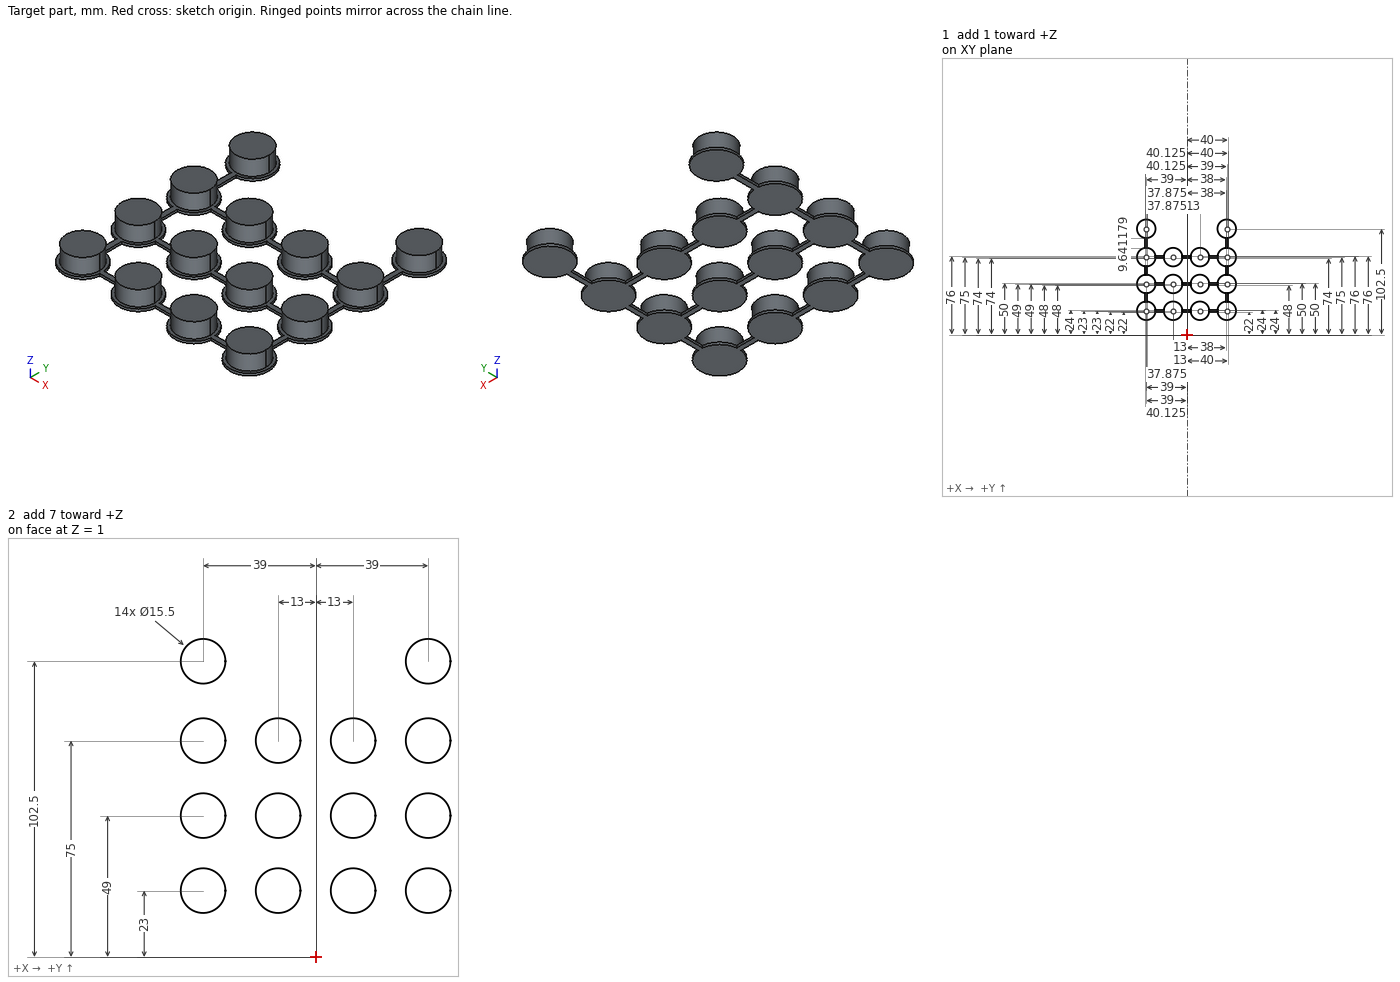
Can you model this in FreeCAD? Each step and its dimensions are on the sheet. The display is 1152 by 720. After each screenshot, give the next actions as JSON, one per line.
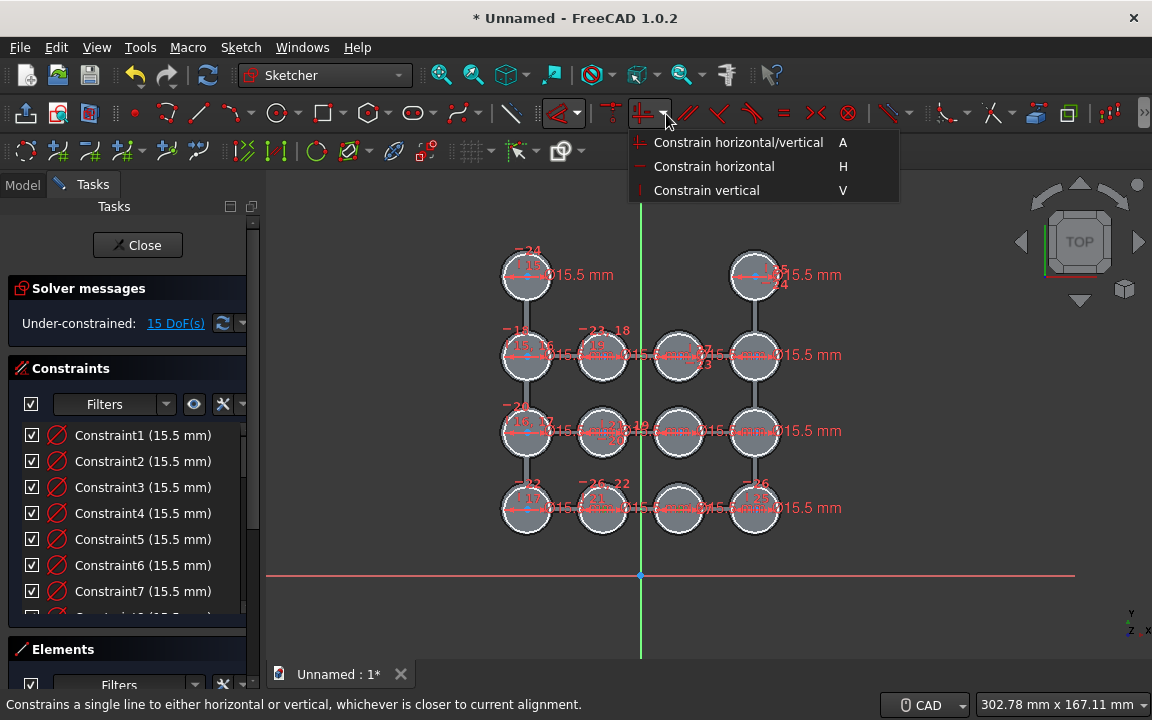
{"action": "left_click", "coordinate": [764, 166]}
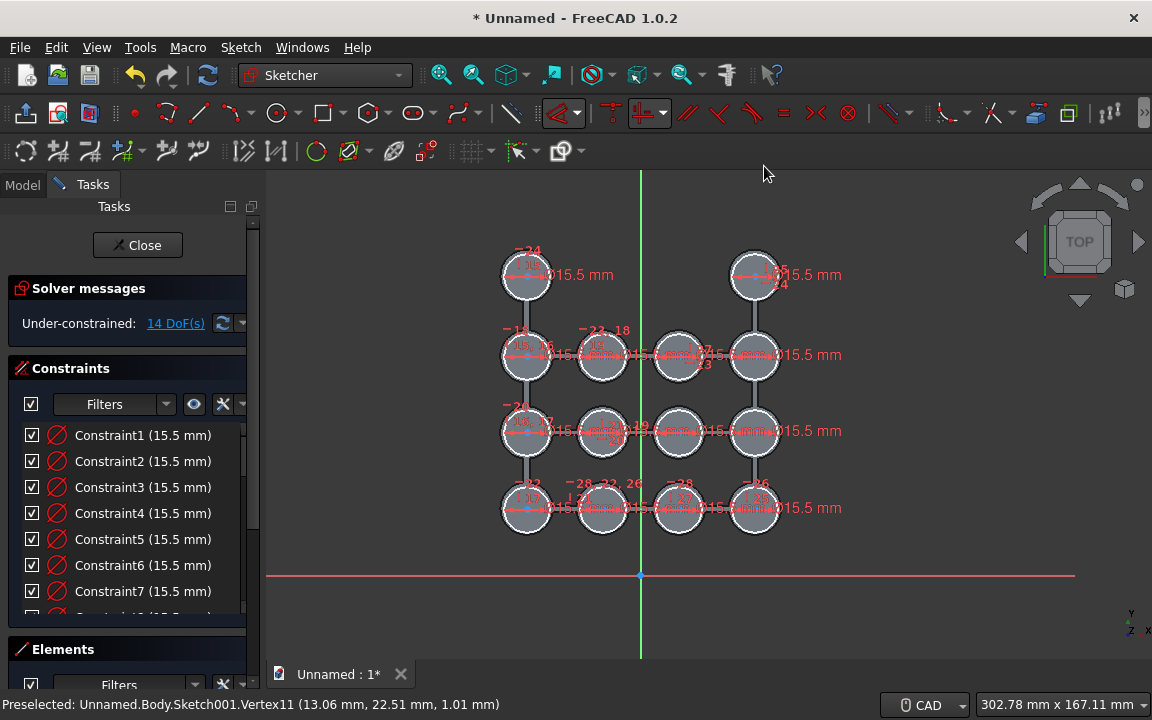
{"action": "left_click", "coordinate": [755, 510]}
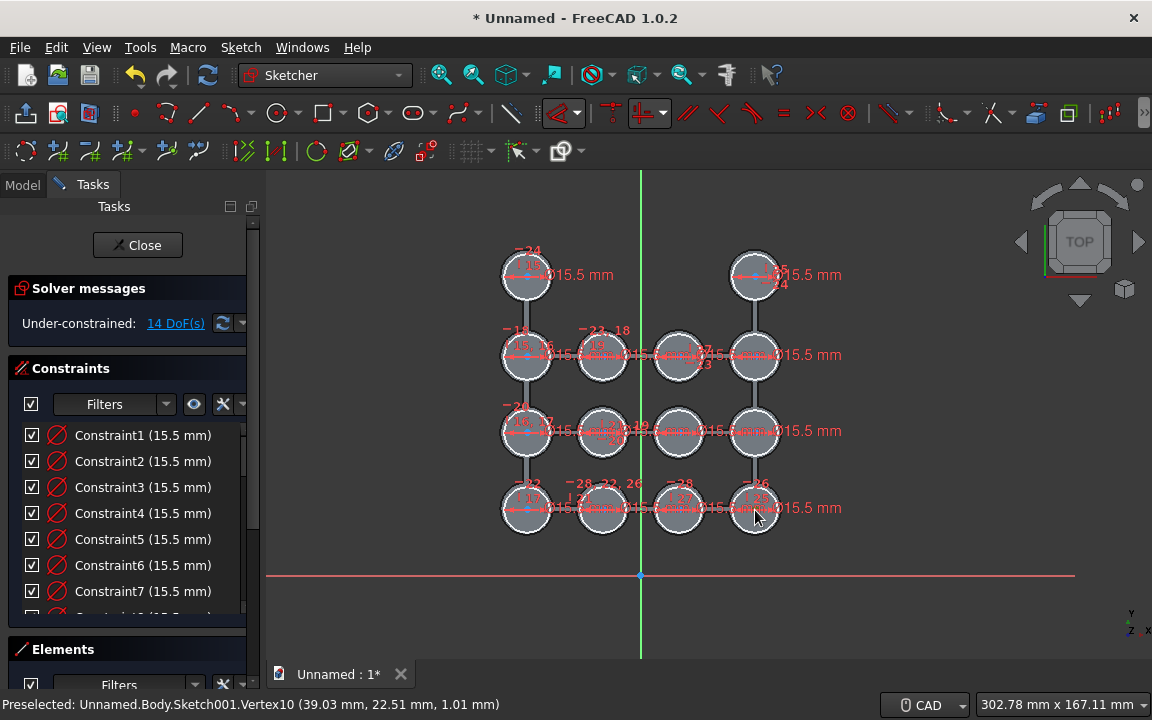
{"action": "left_click", "coordinate": [755, 433]}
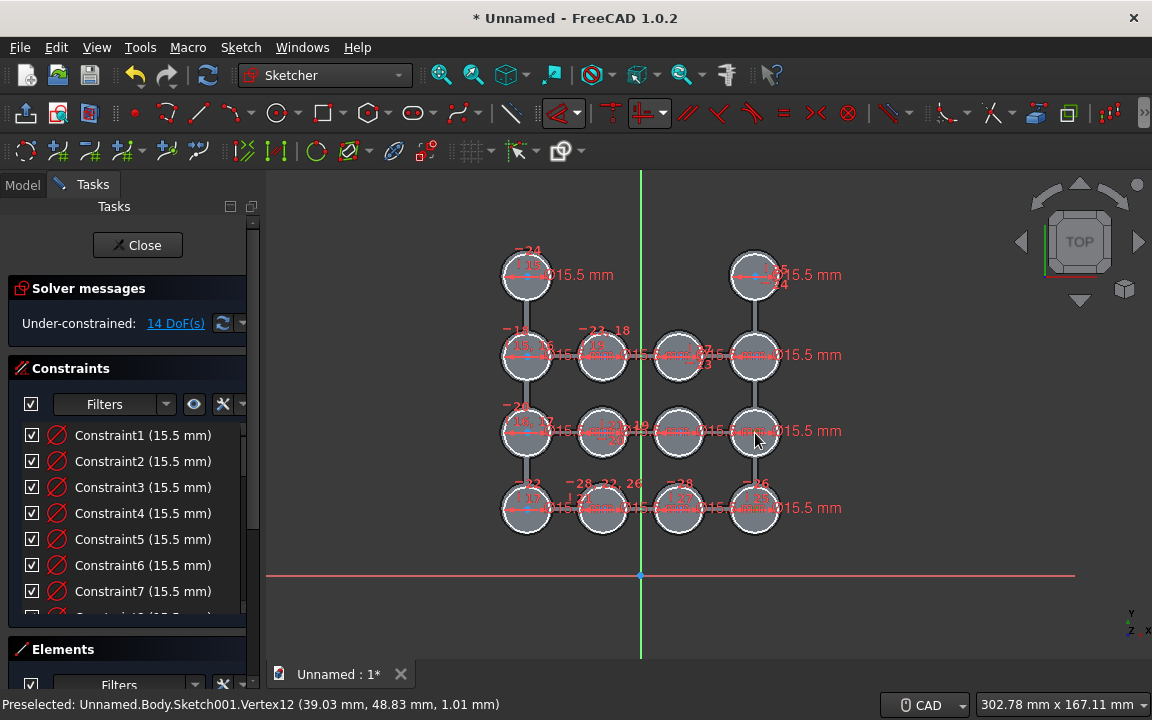
{"action": "left_click", "coordinate": [666, 114]}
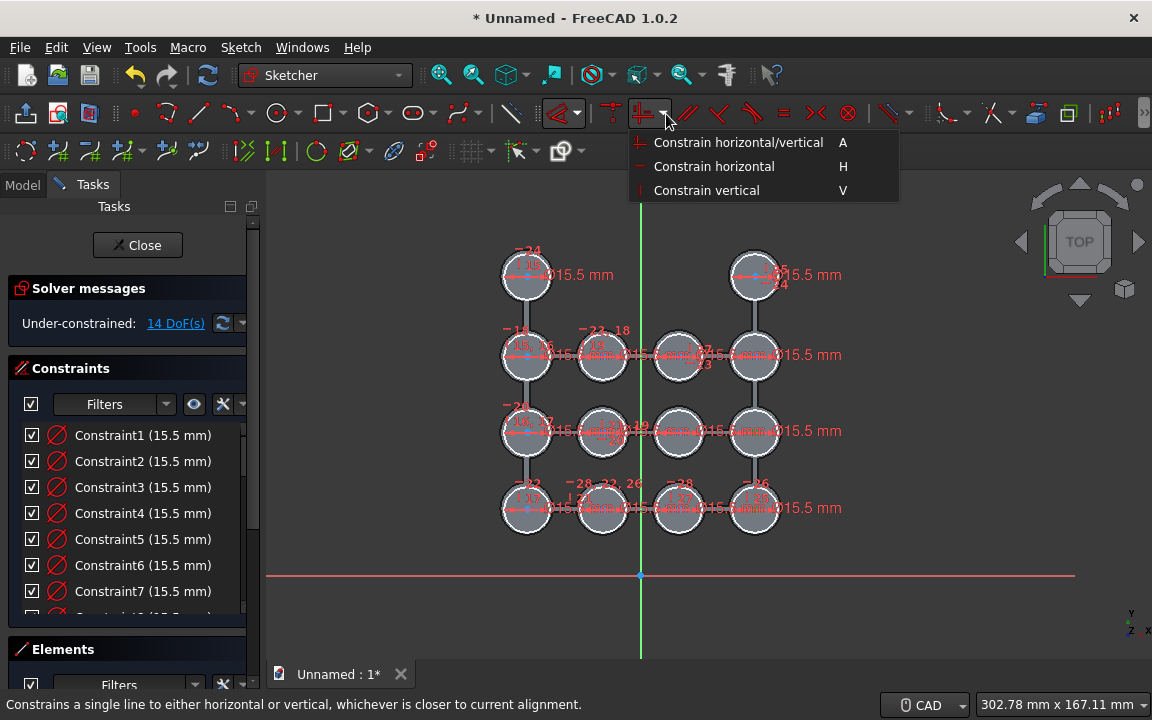
{"action": "left_click", "coordinate": [764, 190]}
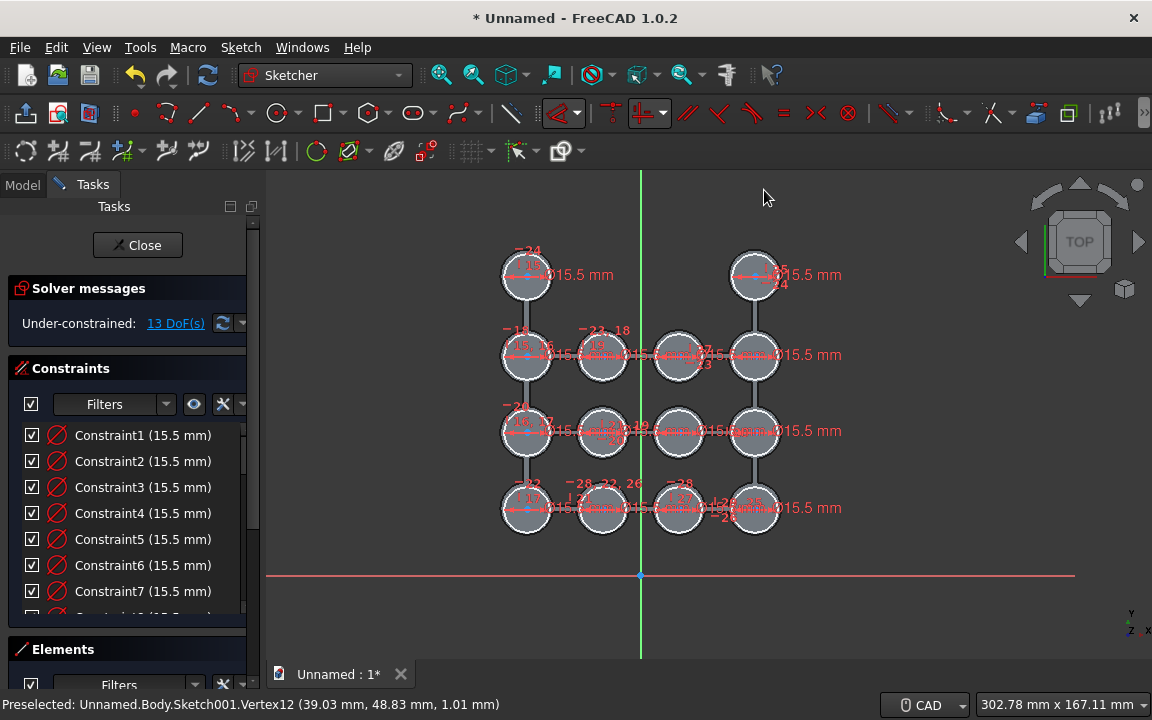
{"action": "left_click", "coordinate": [603, 433]}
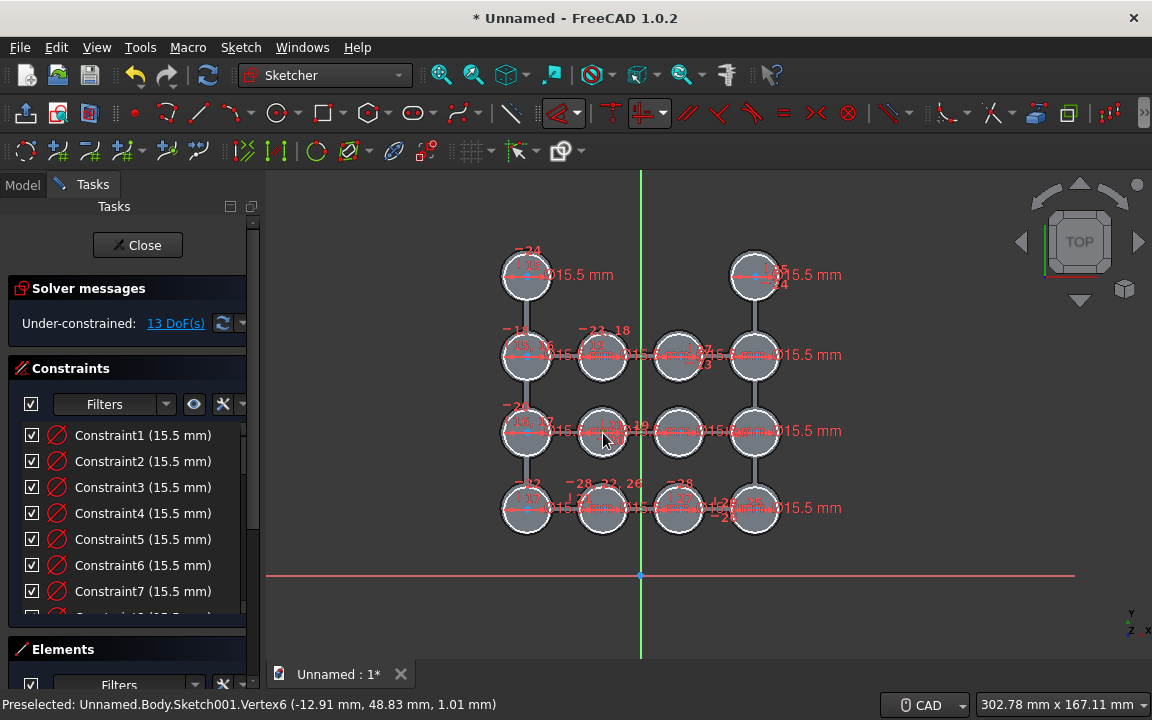
{"action": "left_click", "coordinate": [755, 433]}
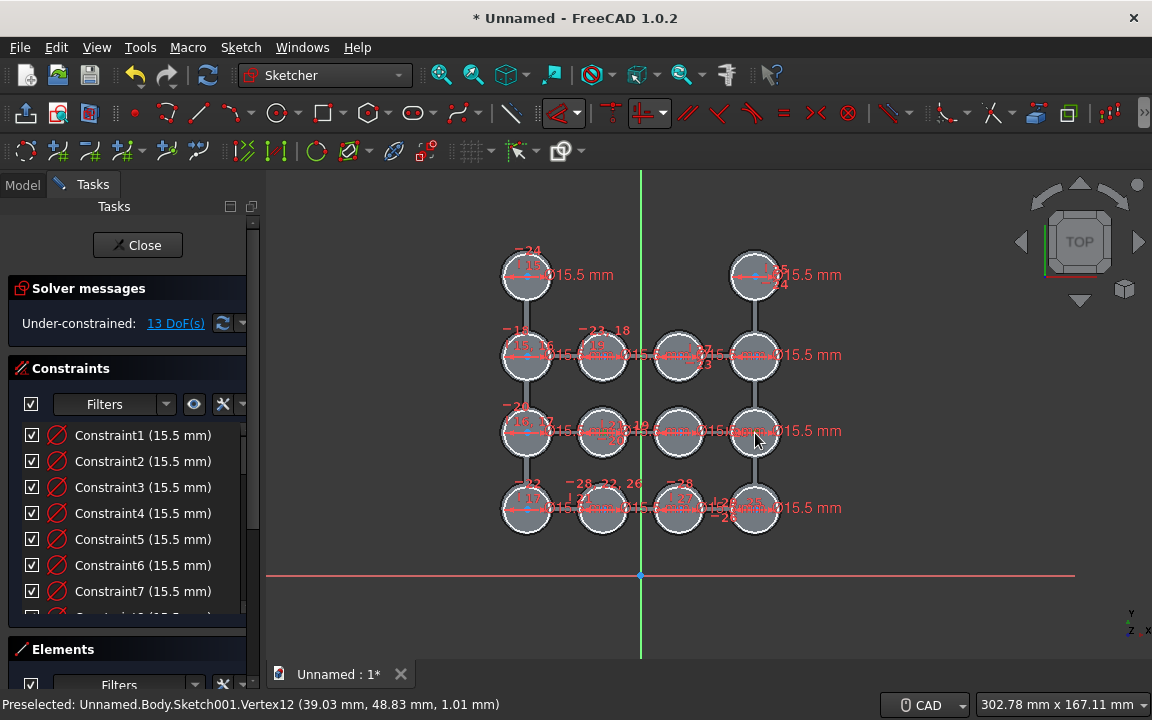
{"action": "key", "text": "h"}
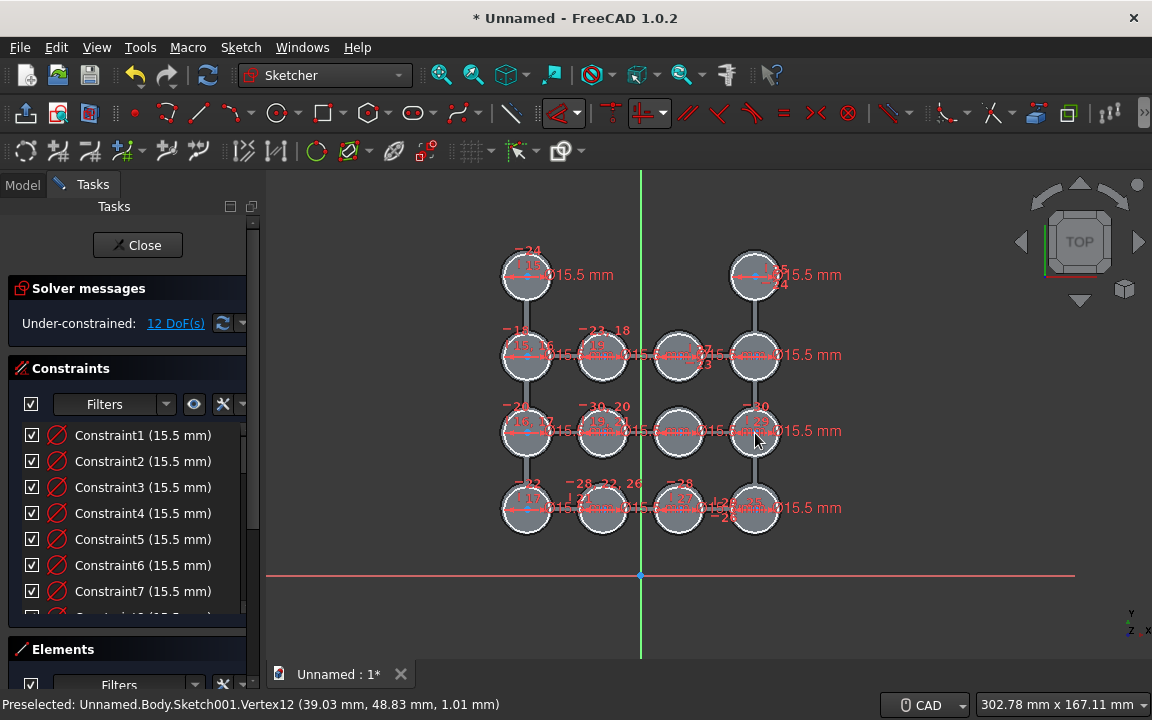
{"action": "left_click", "coordinate": [679, 357]}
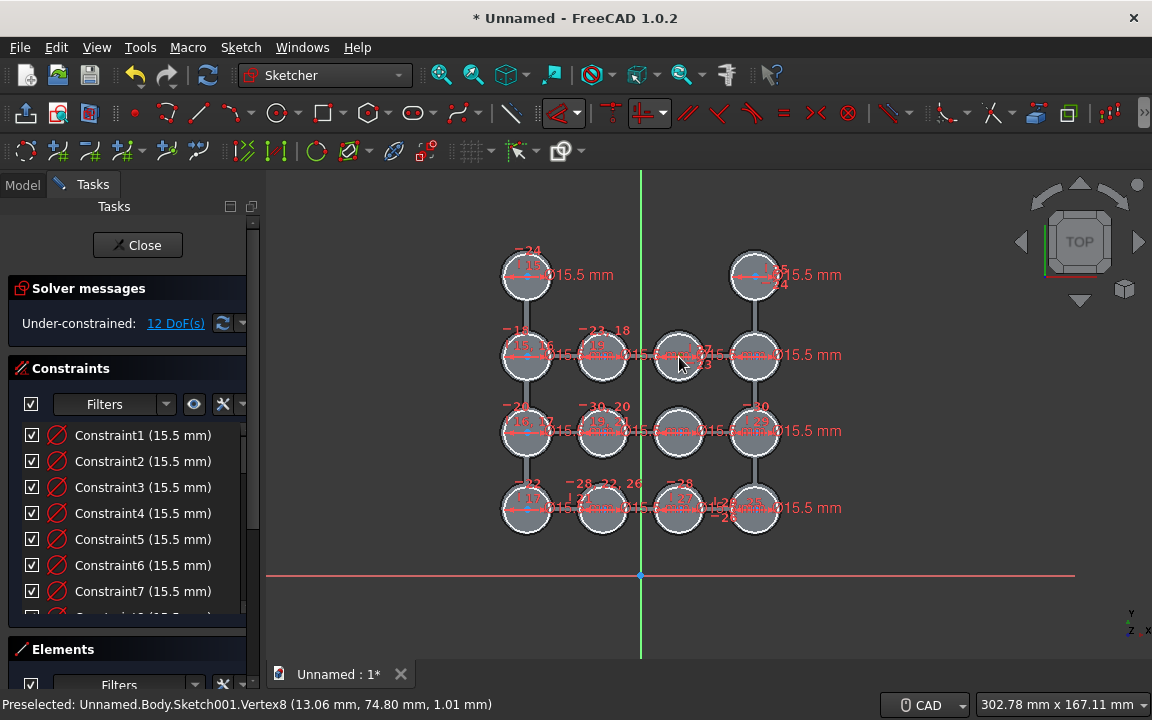
{"action": "left_click", "coordinate": [679, 433]}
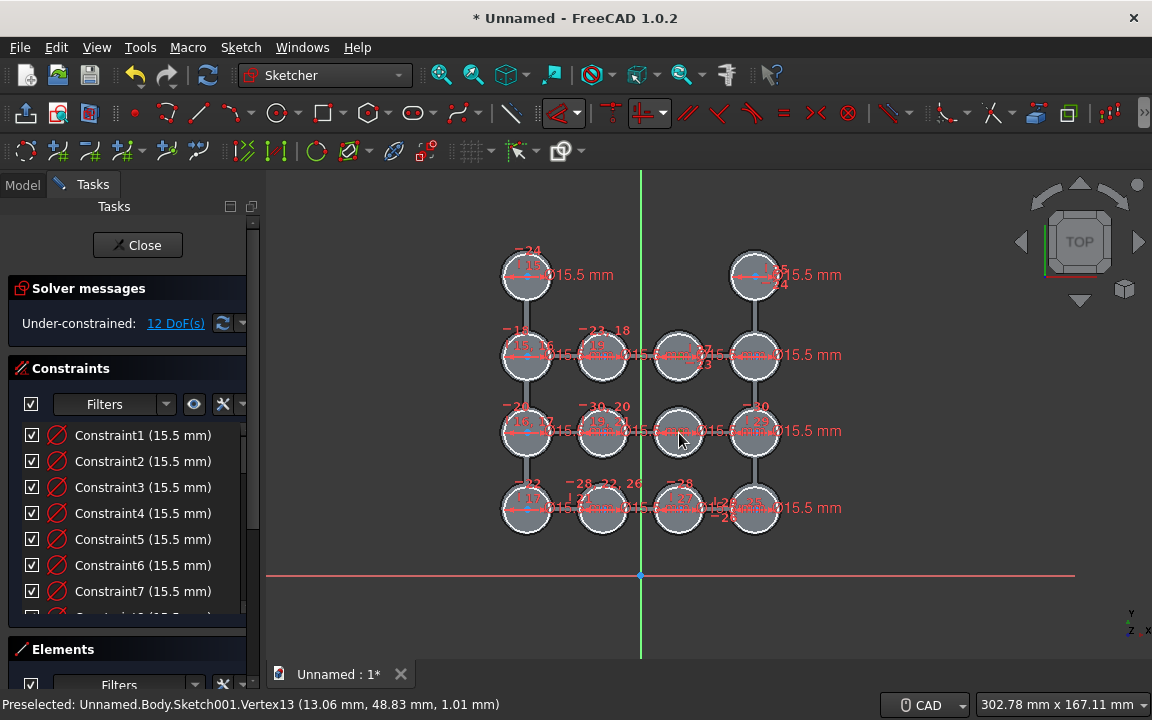
{"action": "key", "text": "v"}